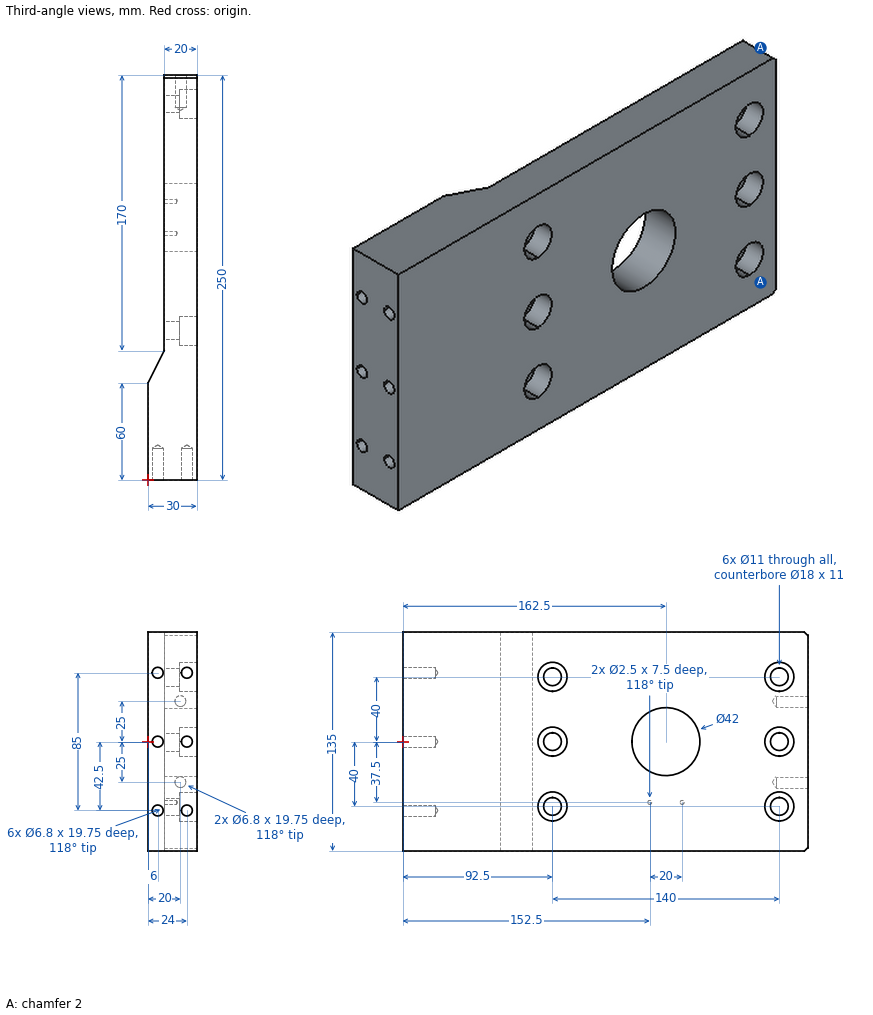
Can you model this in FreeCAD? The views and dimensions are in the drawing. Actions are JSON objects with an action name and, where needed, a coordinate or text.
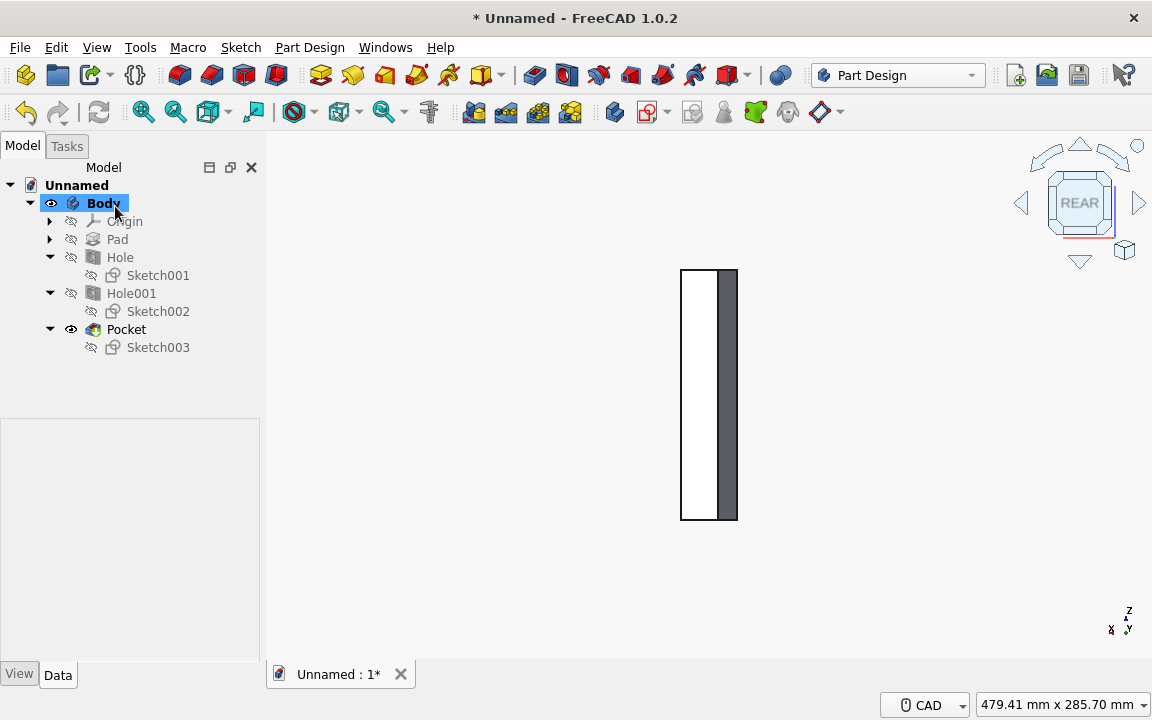
{"action": "left_click", "coordinate": [700, 323]}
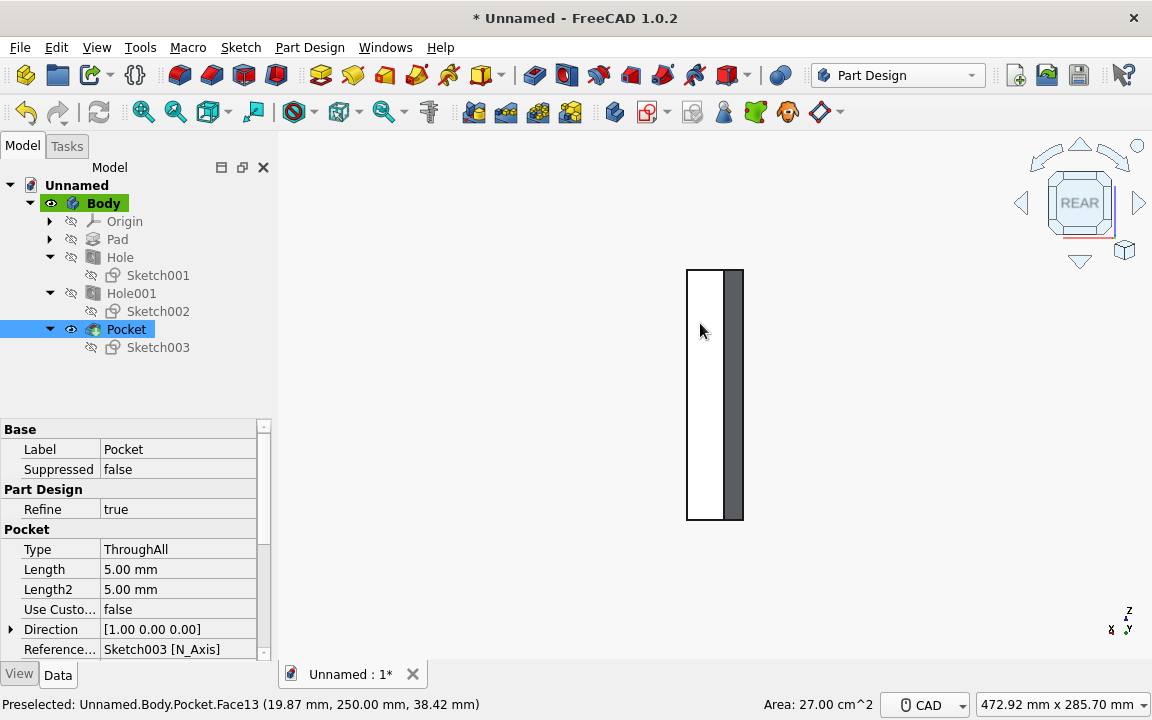
{"action": "left_click", "coordinate": [648, 112]}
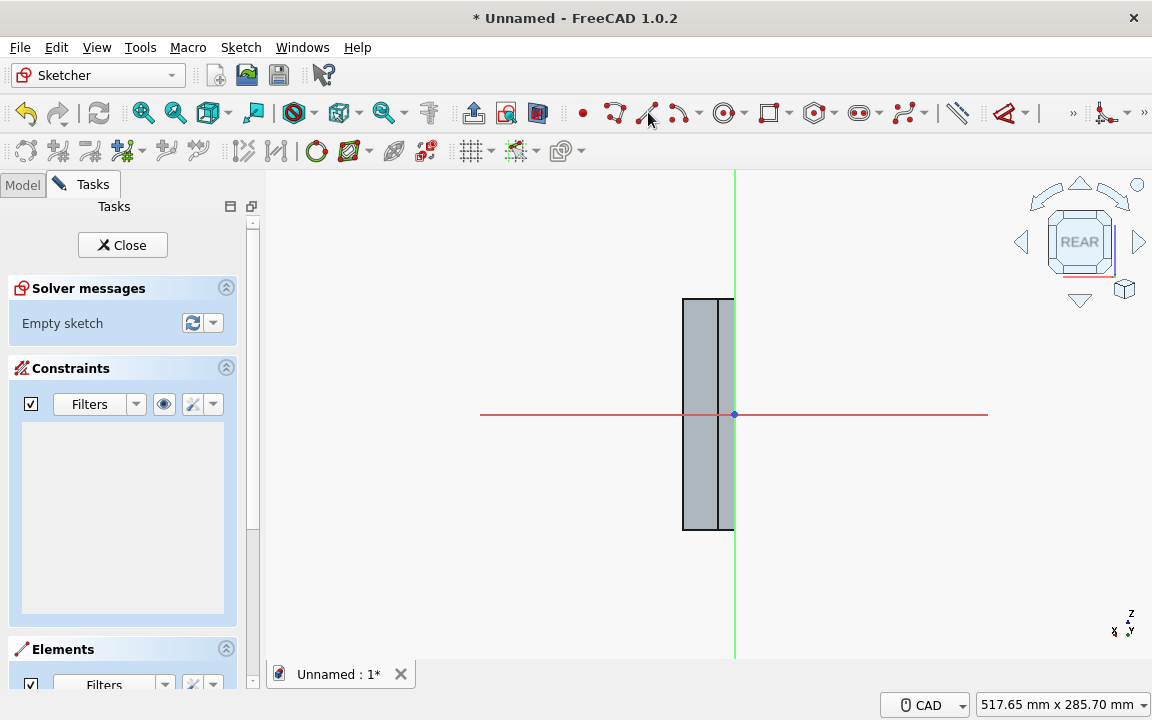
{"action": "scroll", "coordinate": [747, 415], "scroll_direction": "up", "scroll_amount": 6}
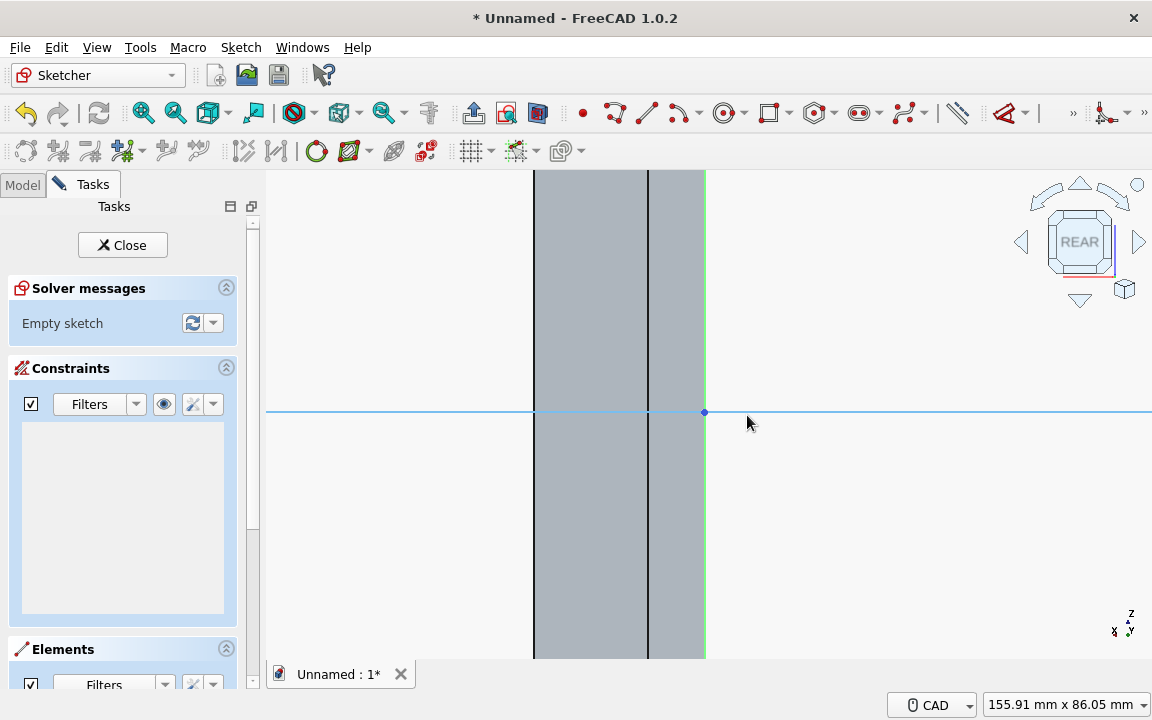
{"action": "left_click", "coordinate": [724, 114]}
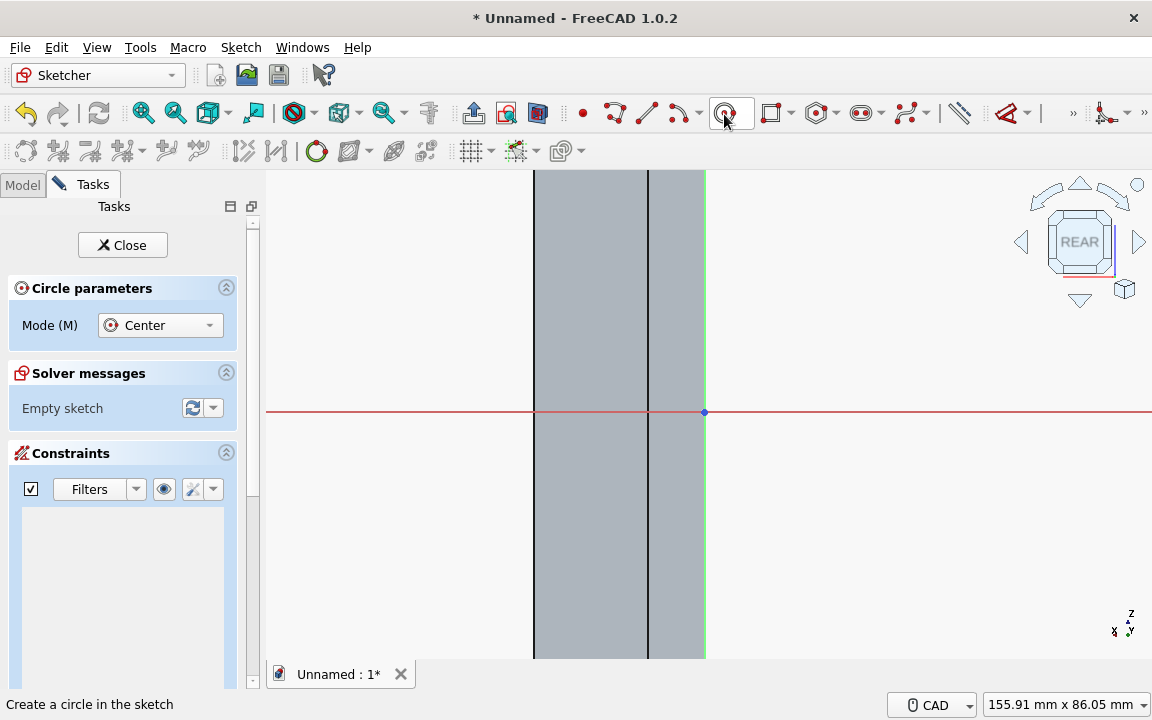
{"action": "left_click", "coordinate": [591, 554]}
{"action": "mouse_move", "coordinate": [605, 541]}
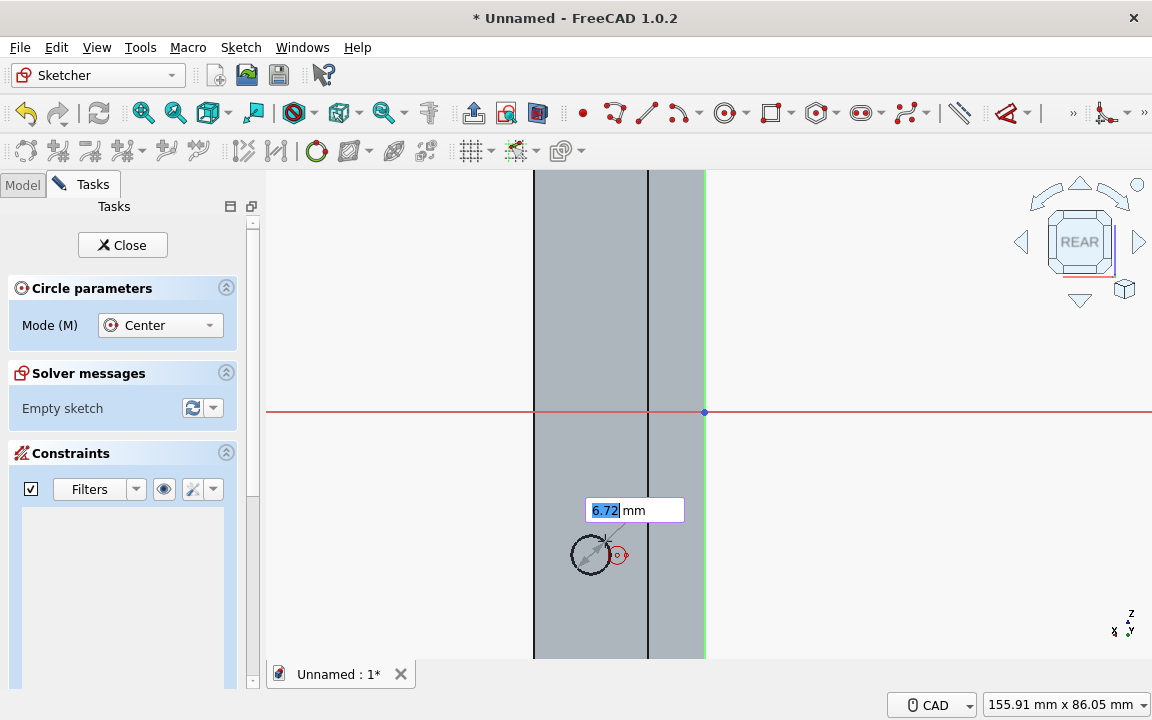
{"action": "type", "text": "6.8"}
{"action": "key", "text": "Return"}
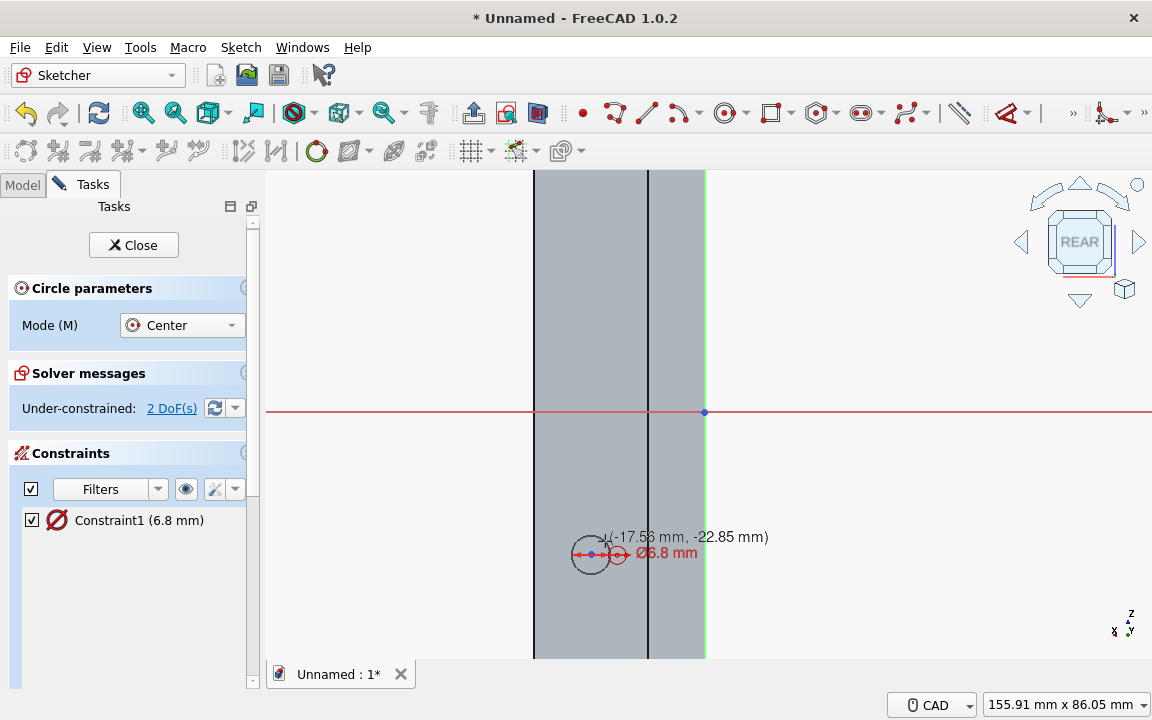
{"action": "left_click", "coordinate": [591, 270]}
{"action": "mouse_move", "coordinate": [605, 256]}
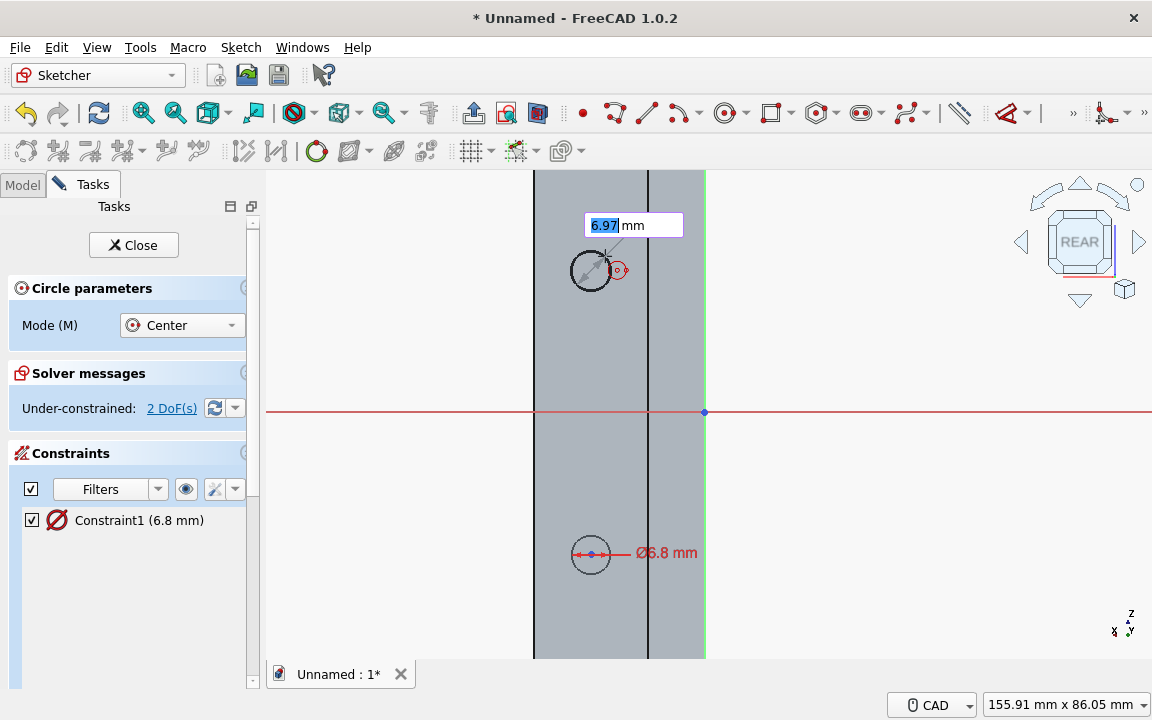
{"action": "type", "text": "6.8"}
{"action": "key", "text": "Return"}
{"action": "key", "text": "Escape"}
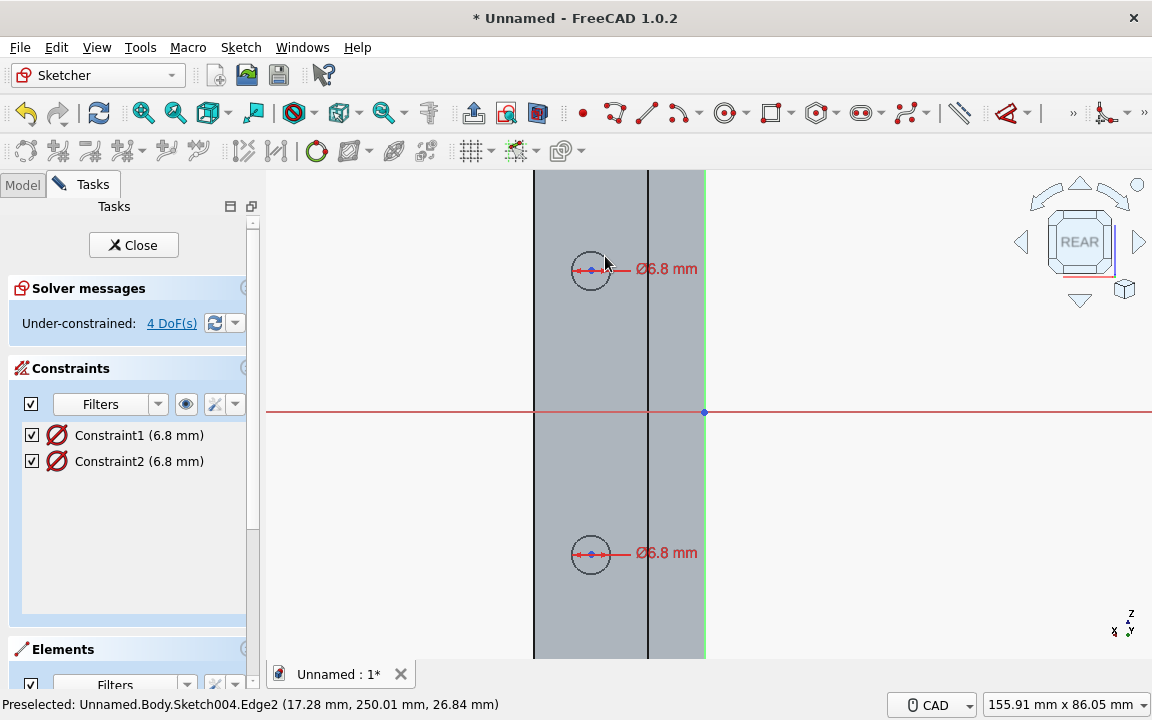
{"action": "left_click", "coordinate": [591, 555]}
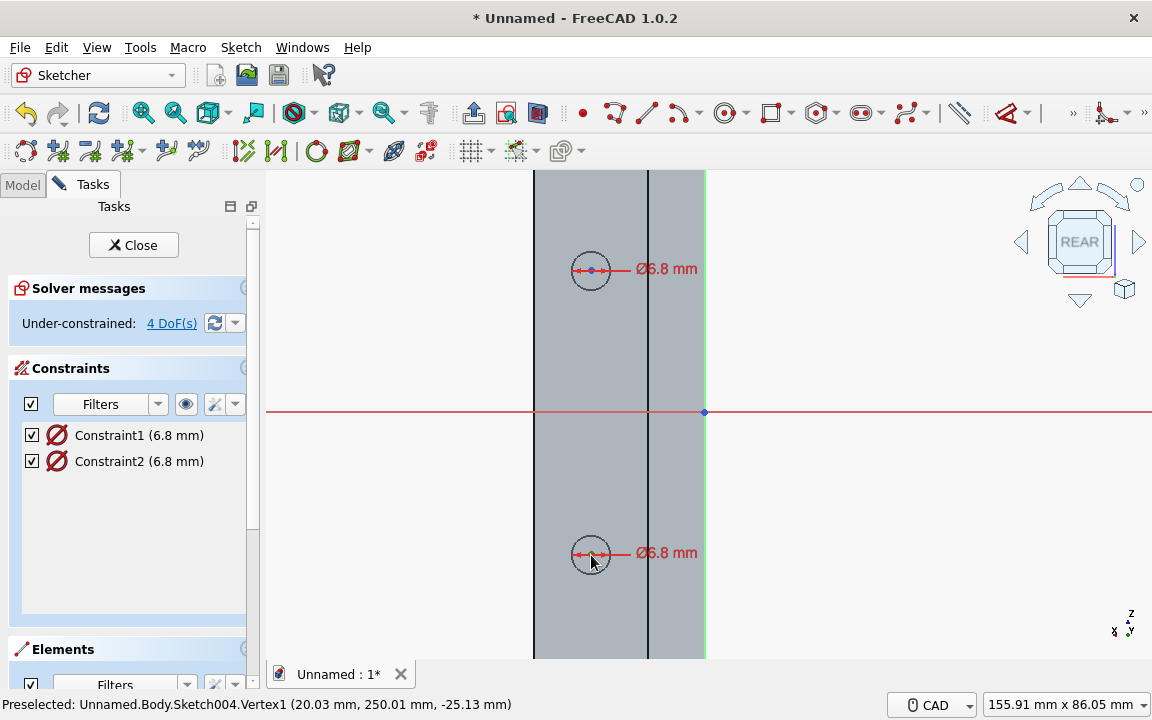
{"action": "left_click", "coordinate": [591, 271]}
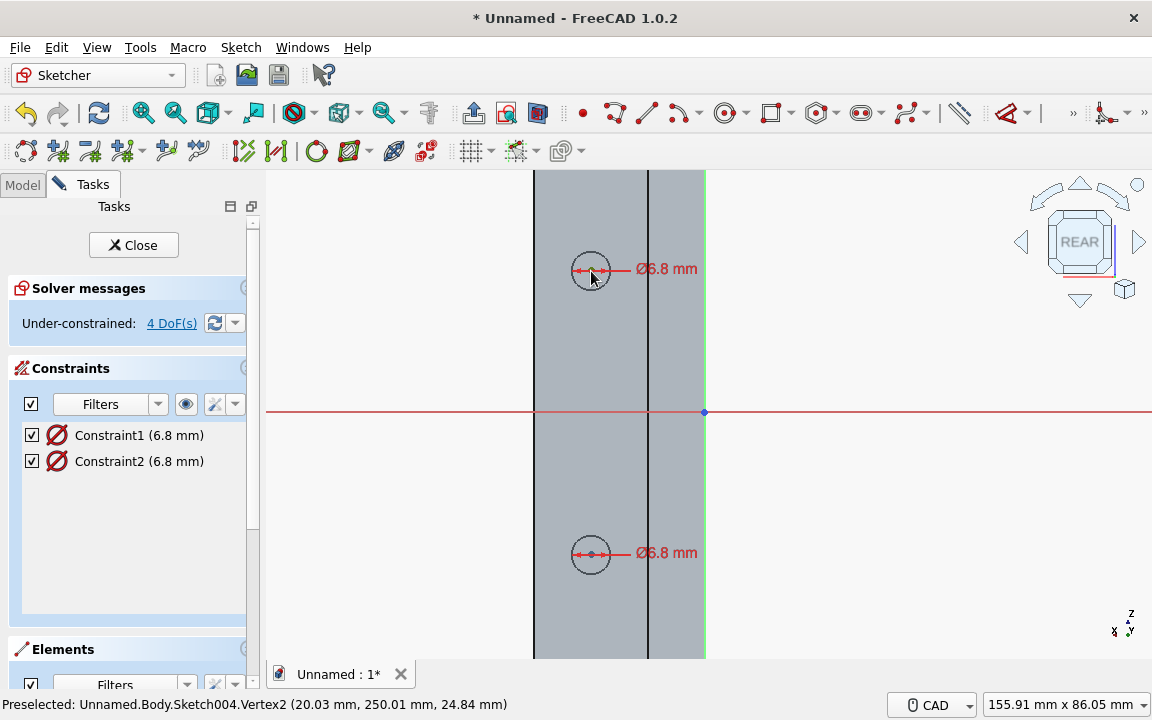
{"action": "key", "text": "v"}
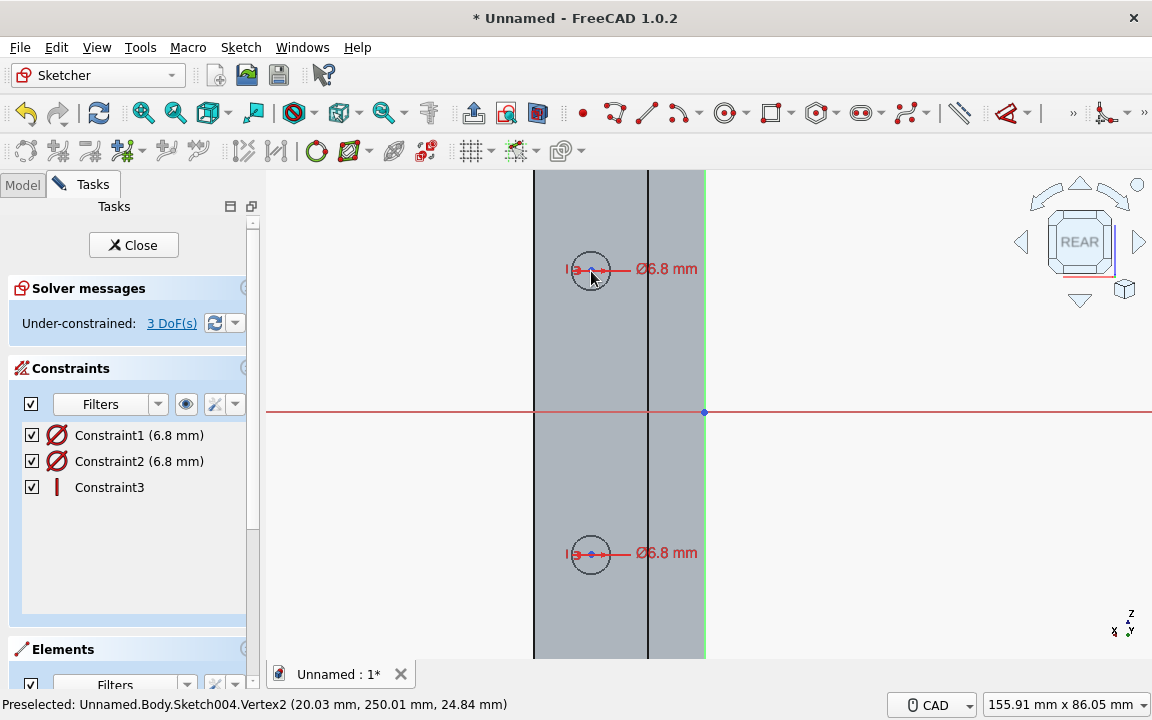
{"action": "left_click", "coordinate": [1006, 114]}